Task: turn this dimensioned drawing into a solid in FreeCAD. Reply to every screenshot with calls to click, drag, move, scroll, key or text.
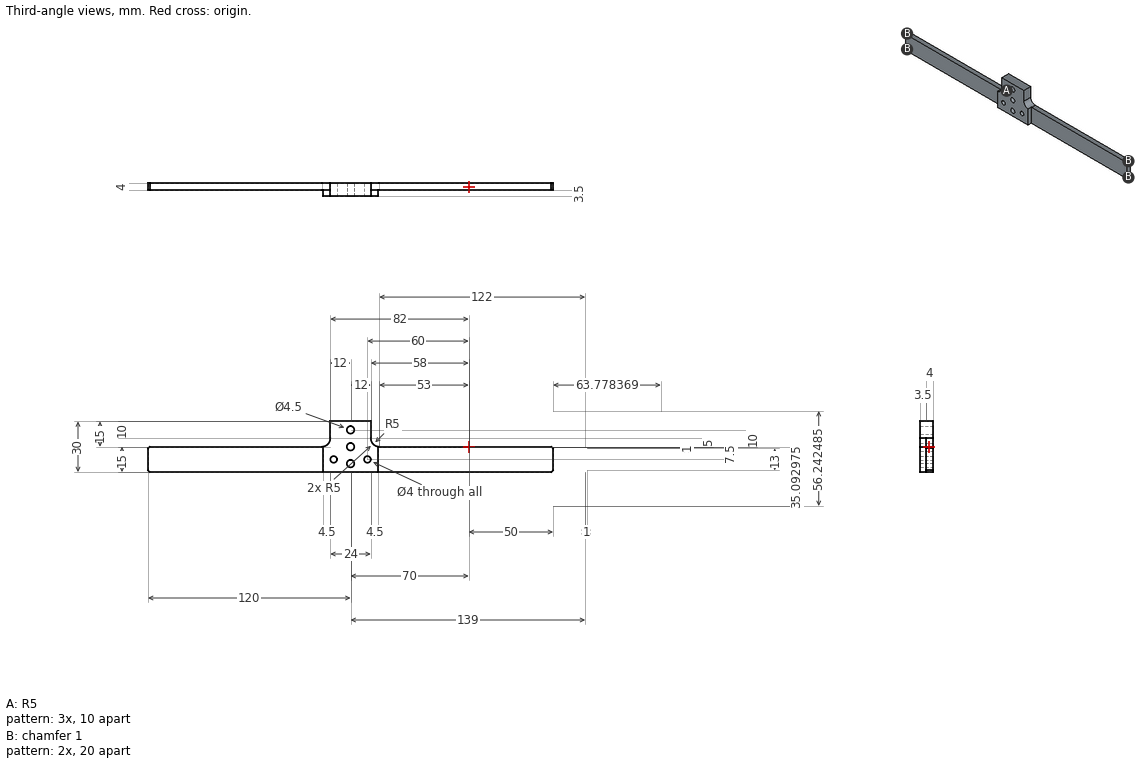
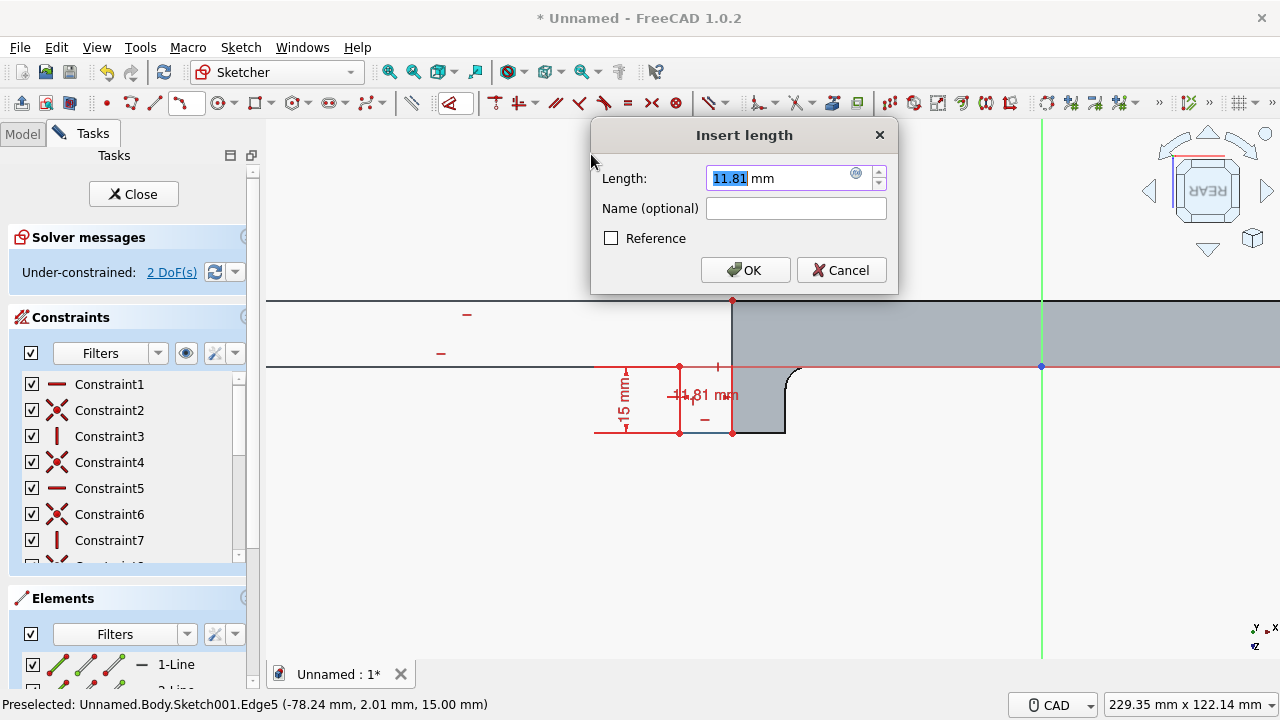
text(12)
key(Return)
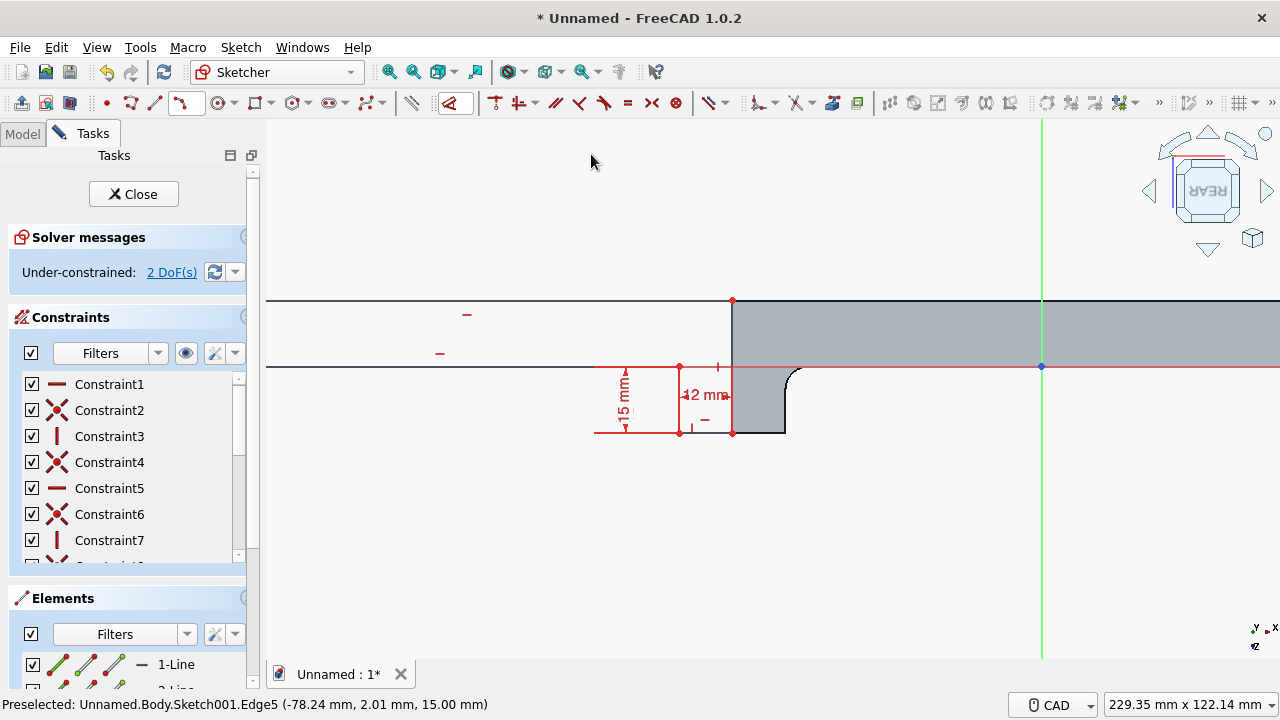
click(573, 301)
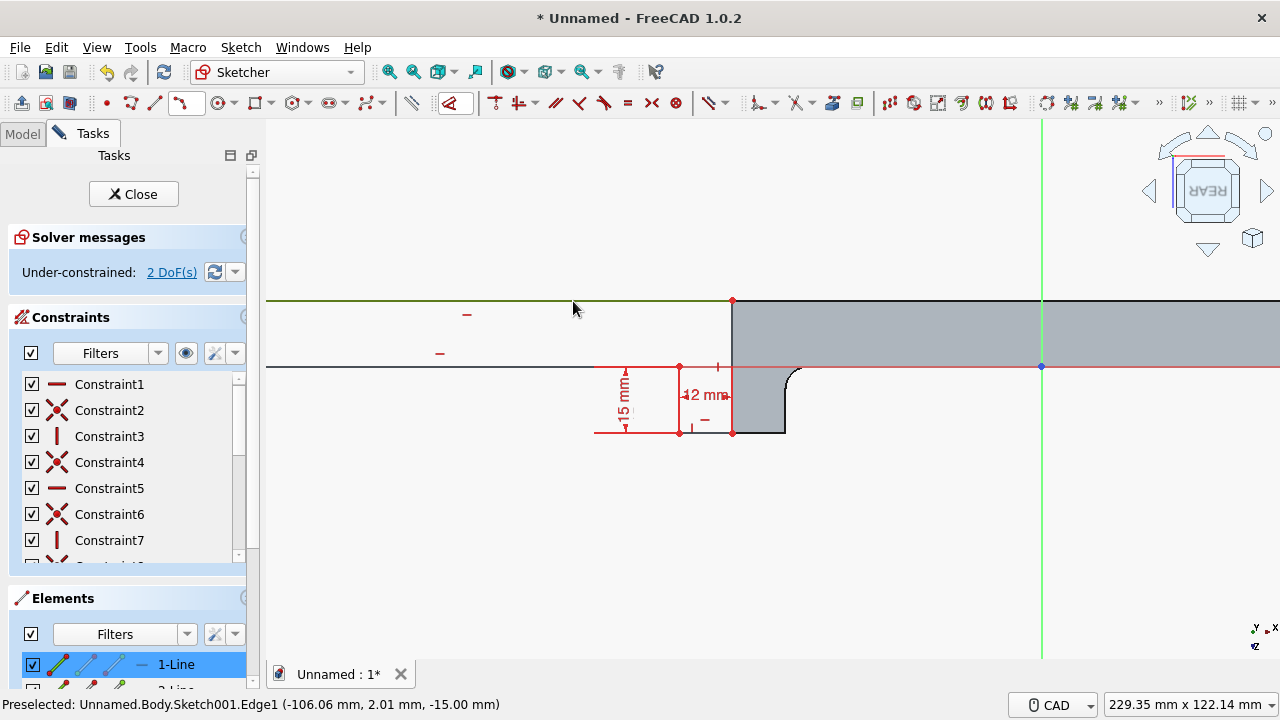
key(l)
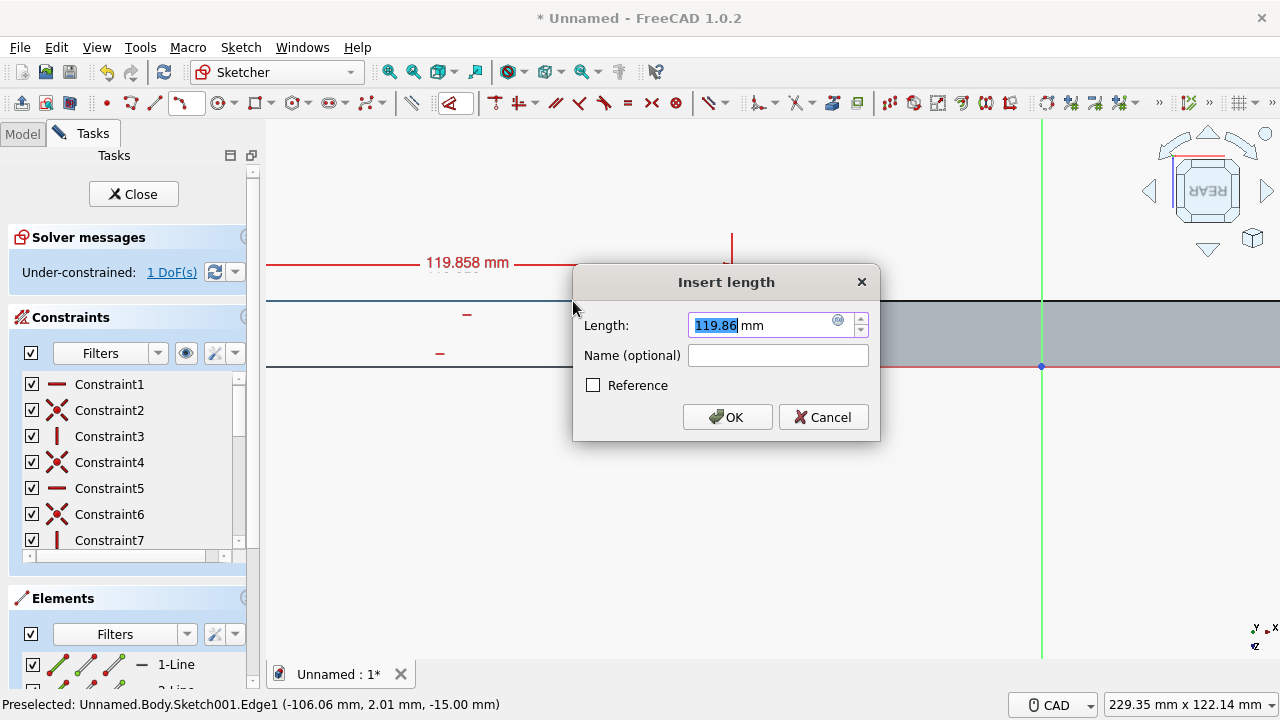
text(120)
key(Return)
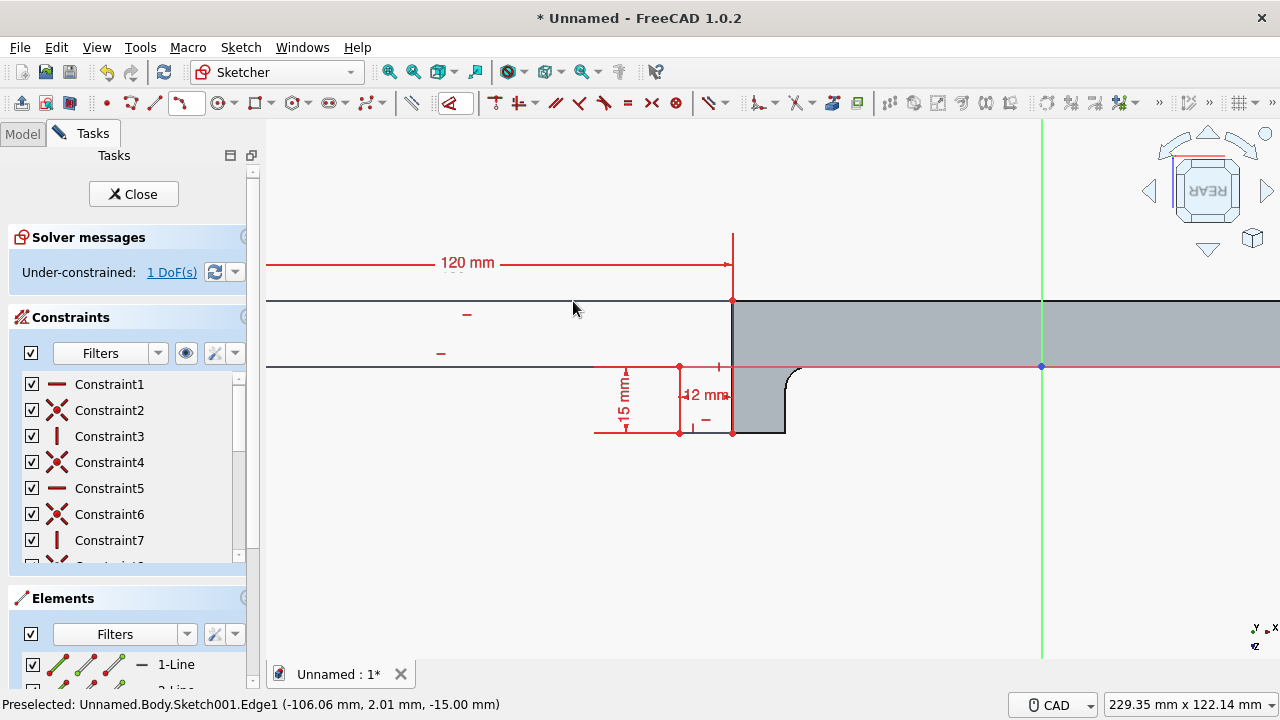
click(733, 301)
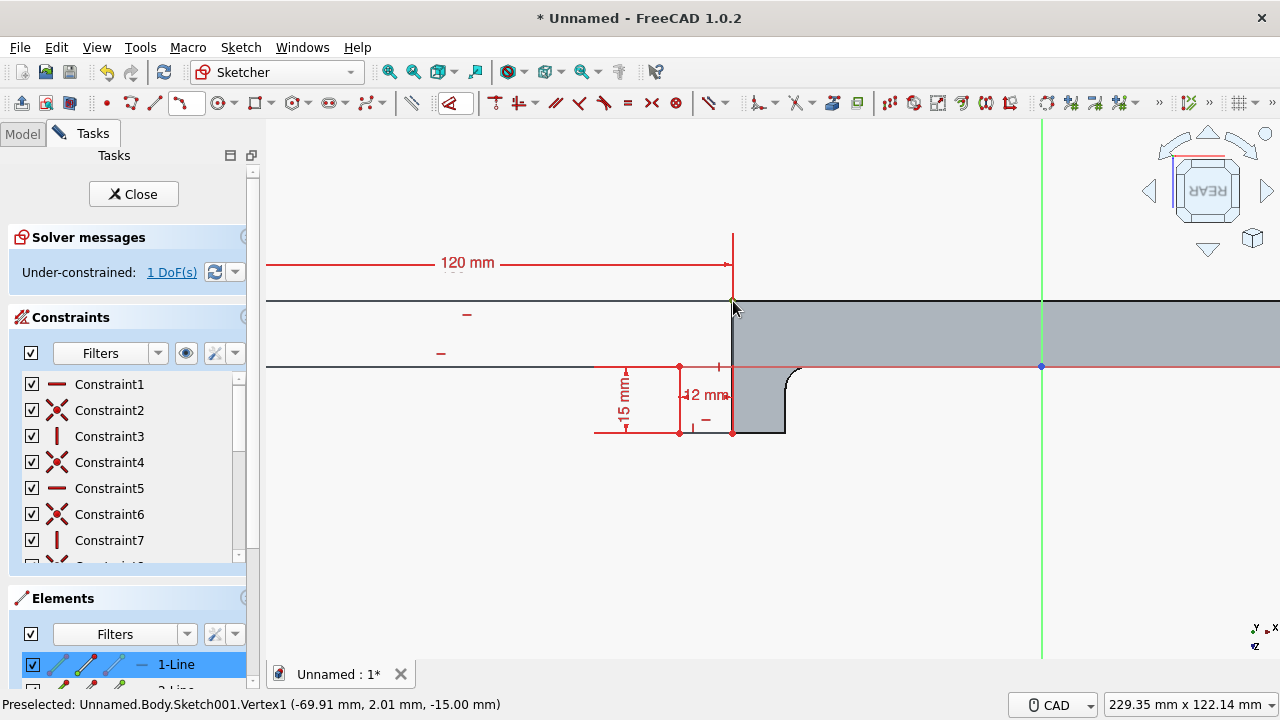
click(468, 104)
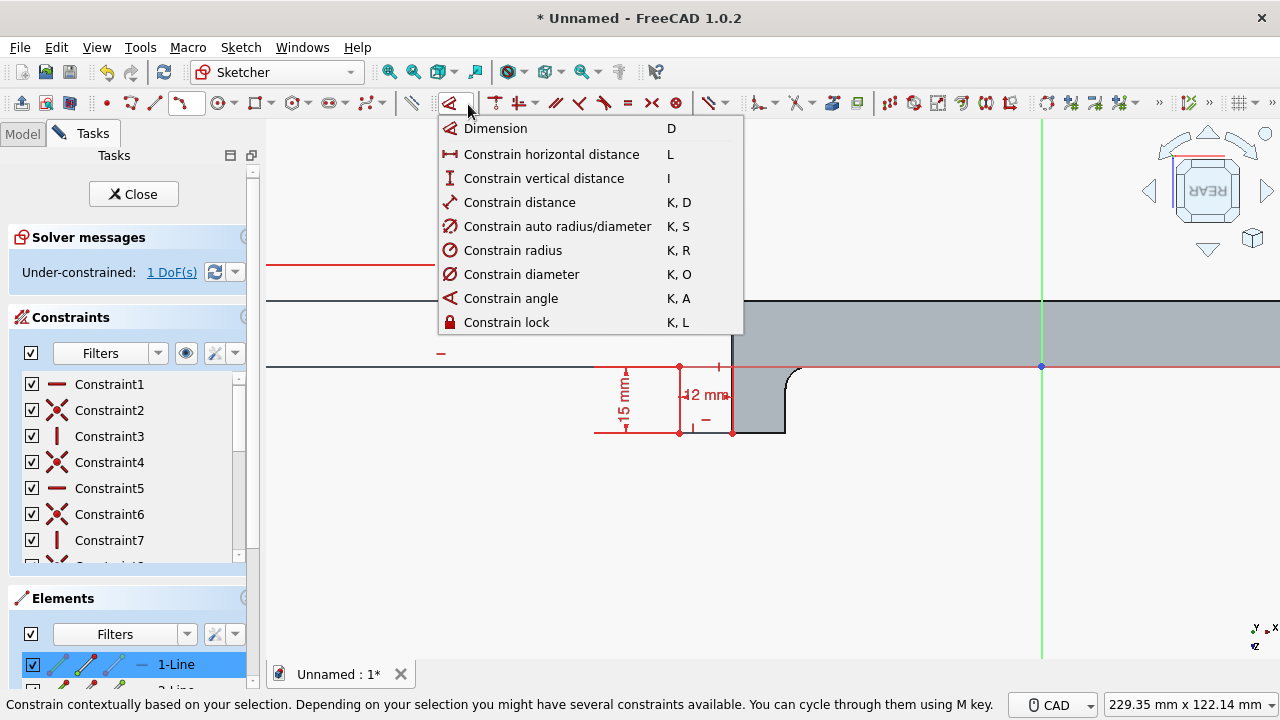
click(591, 154)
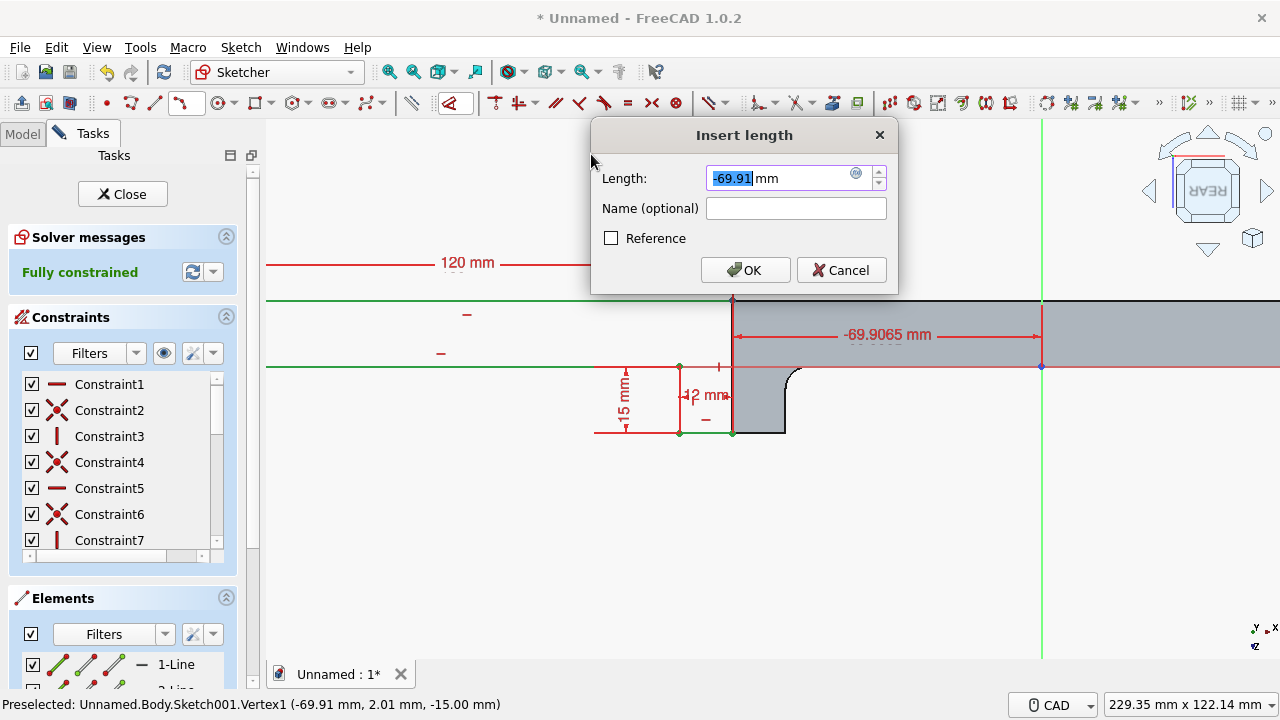
text(-70)
key(Return)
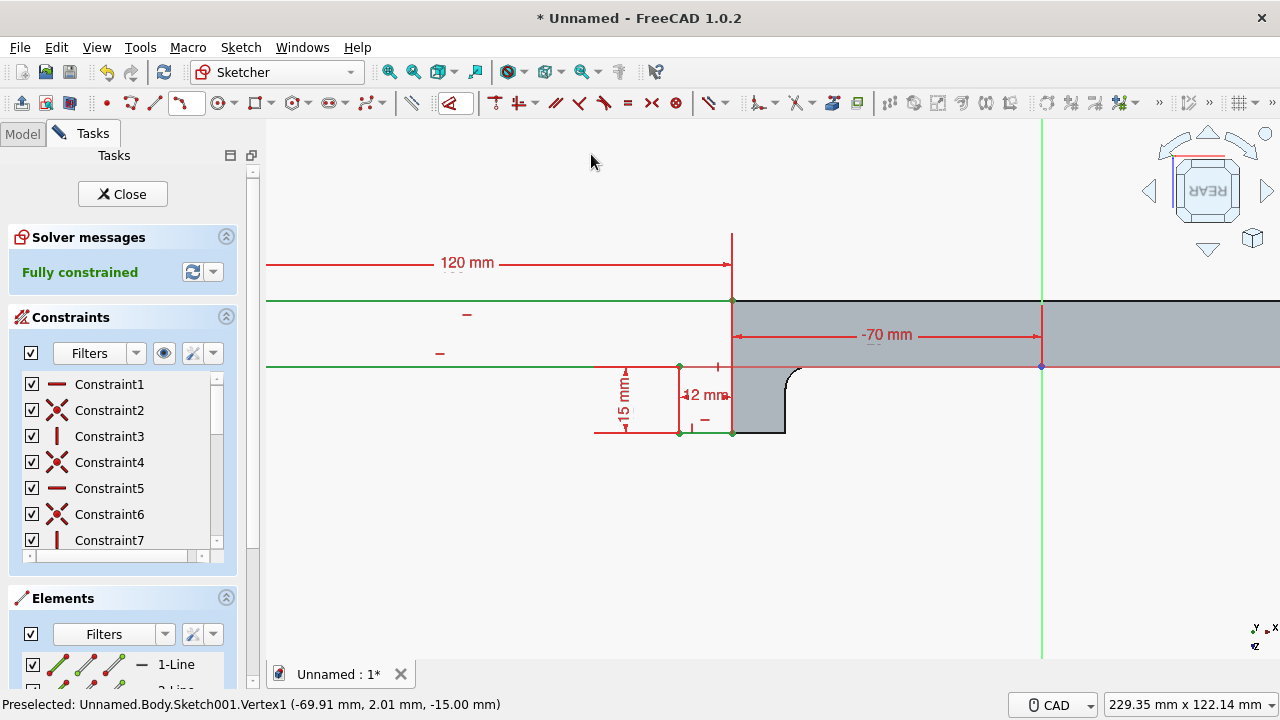
click(123, 194)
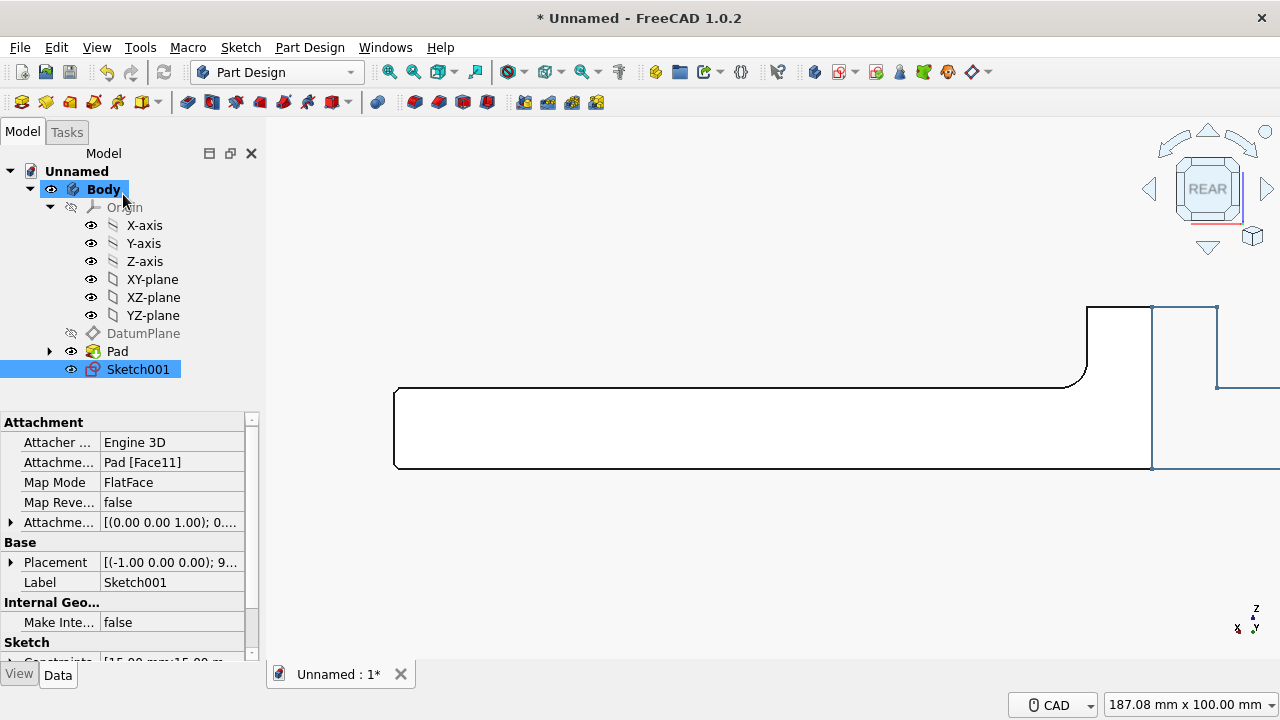
click(22, 102)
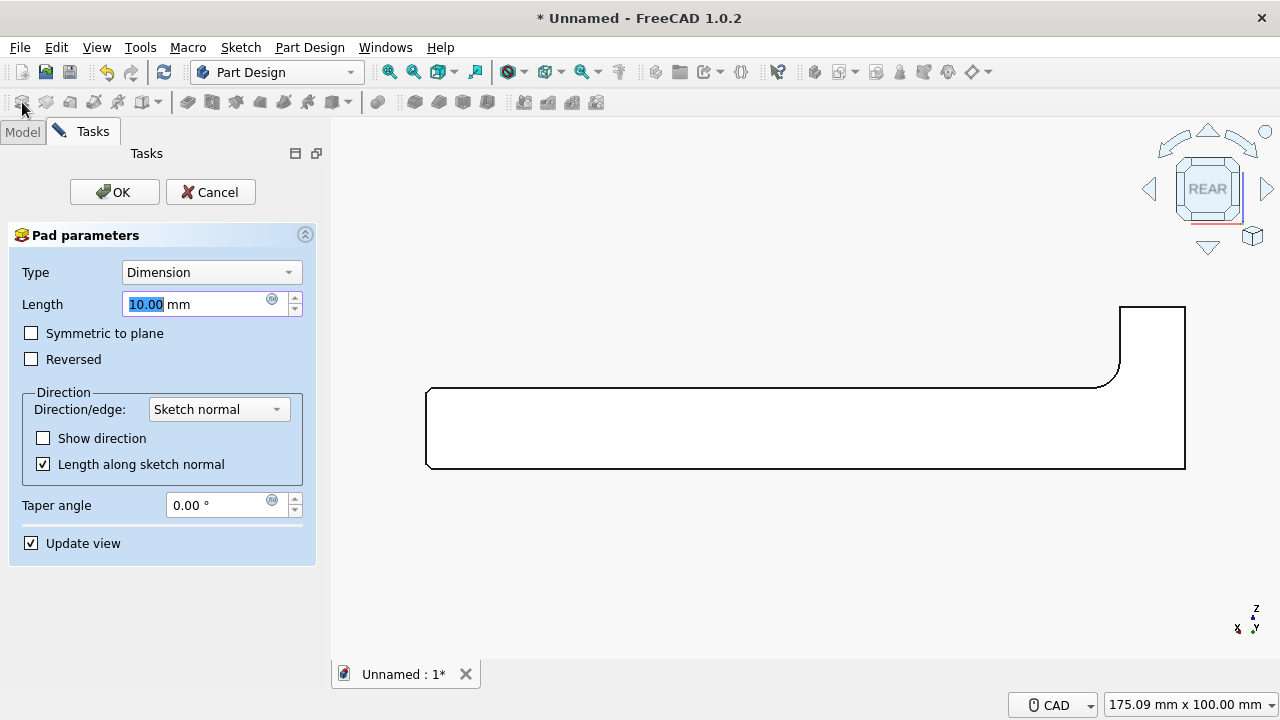
text(4)
key(Tab)